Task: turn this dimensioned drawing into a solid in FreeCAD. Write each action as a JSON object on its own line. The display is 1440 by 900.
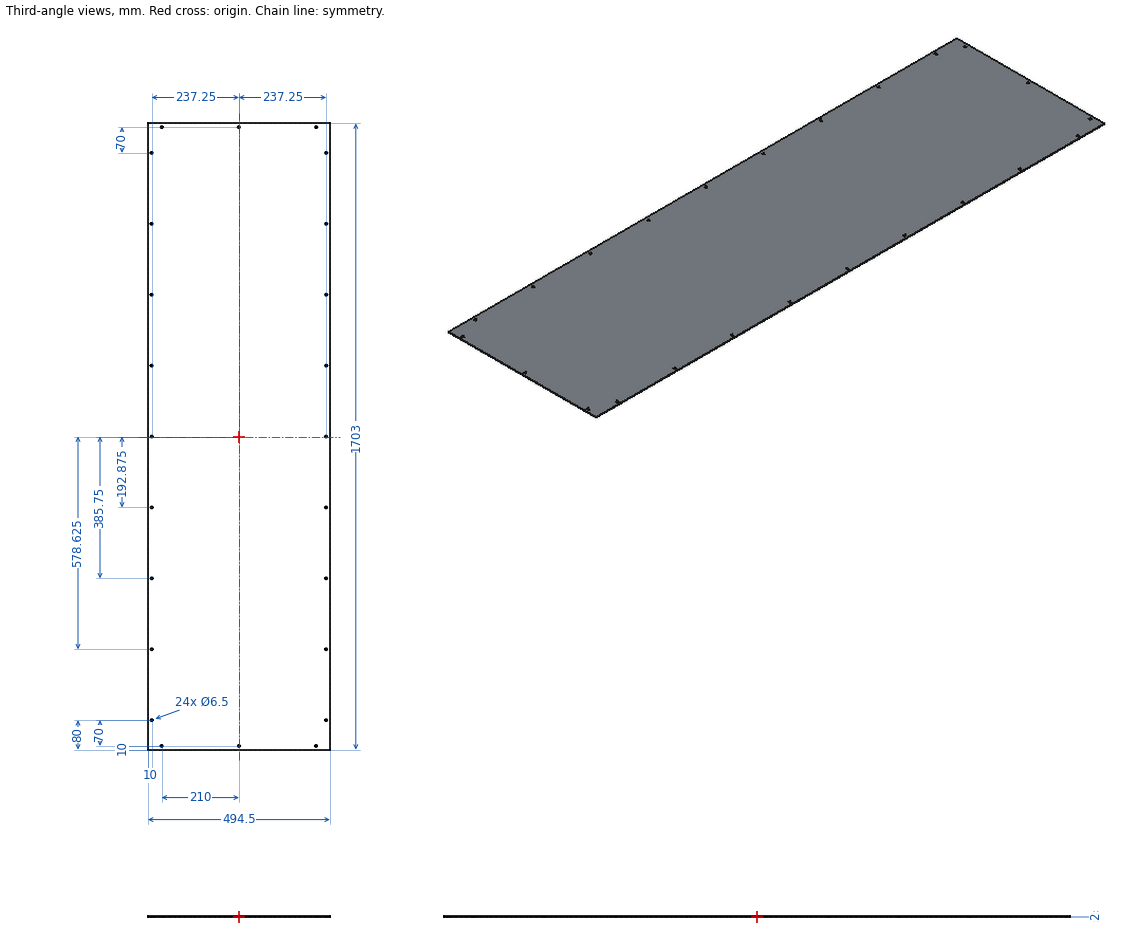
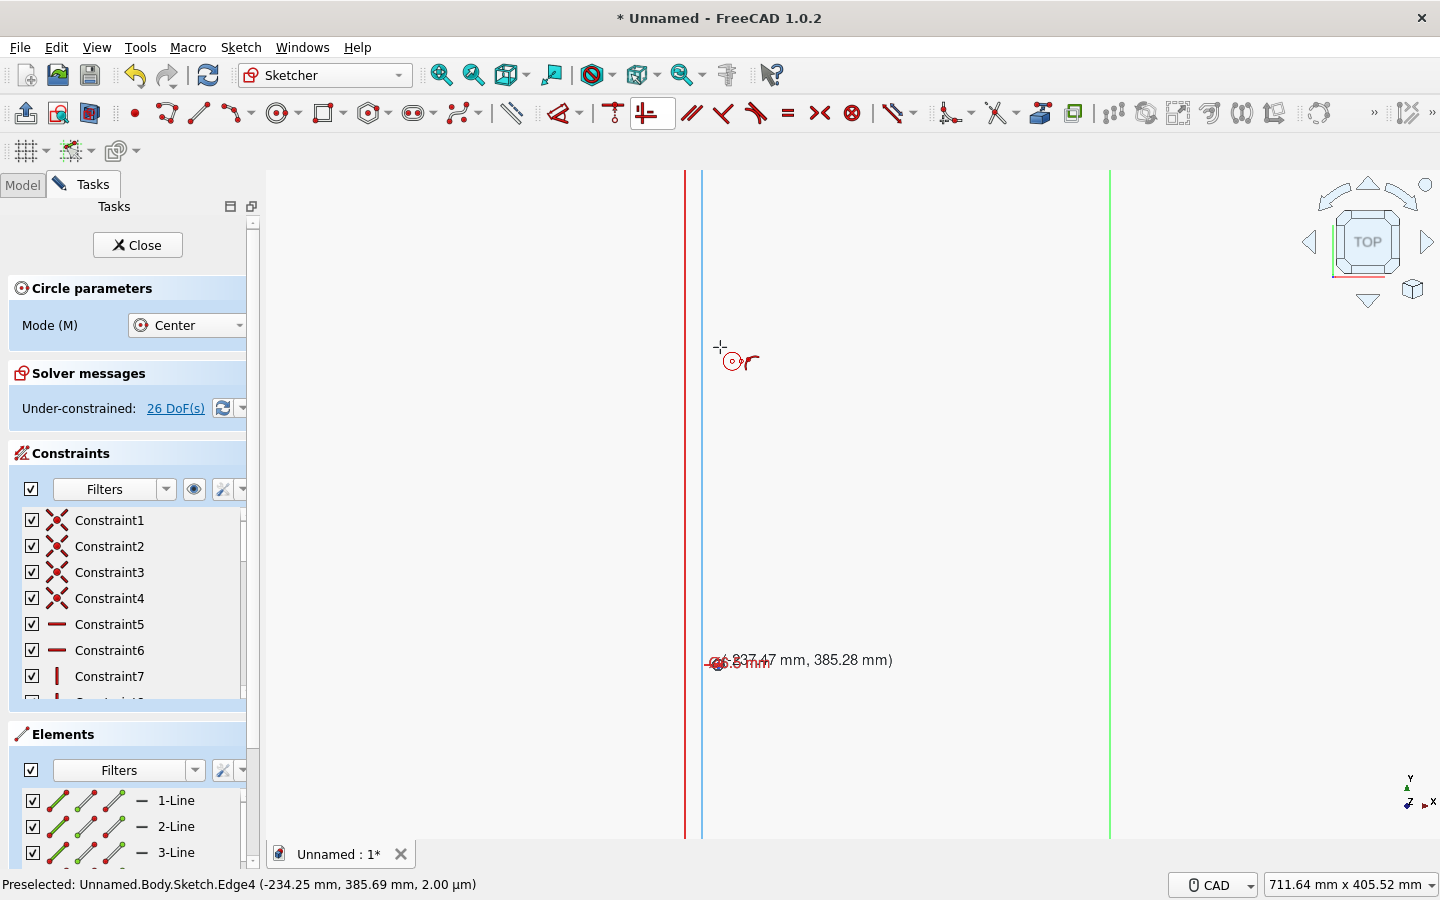
{"action": "left_click", "coordinate": [718, 346]}
{"action": "mouse_move", "coordinate": [722, 342]}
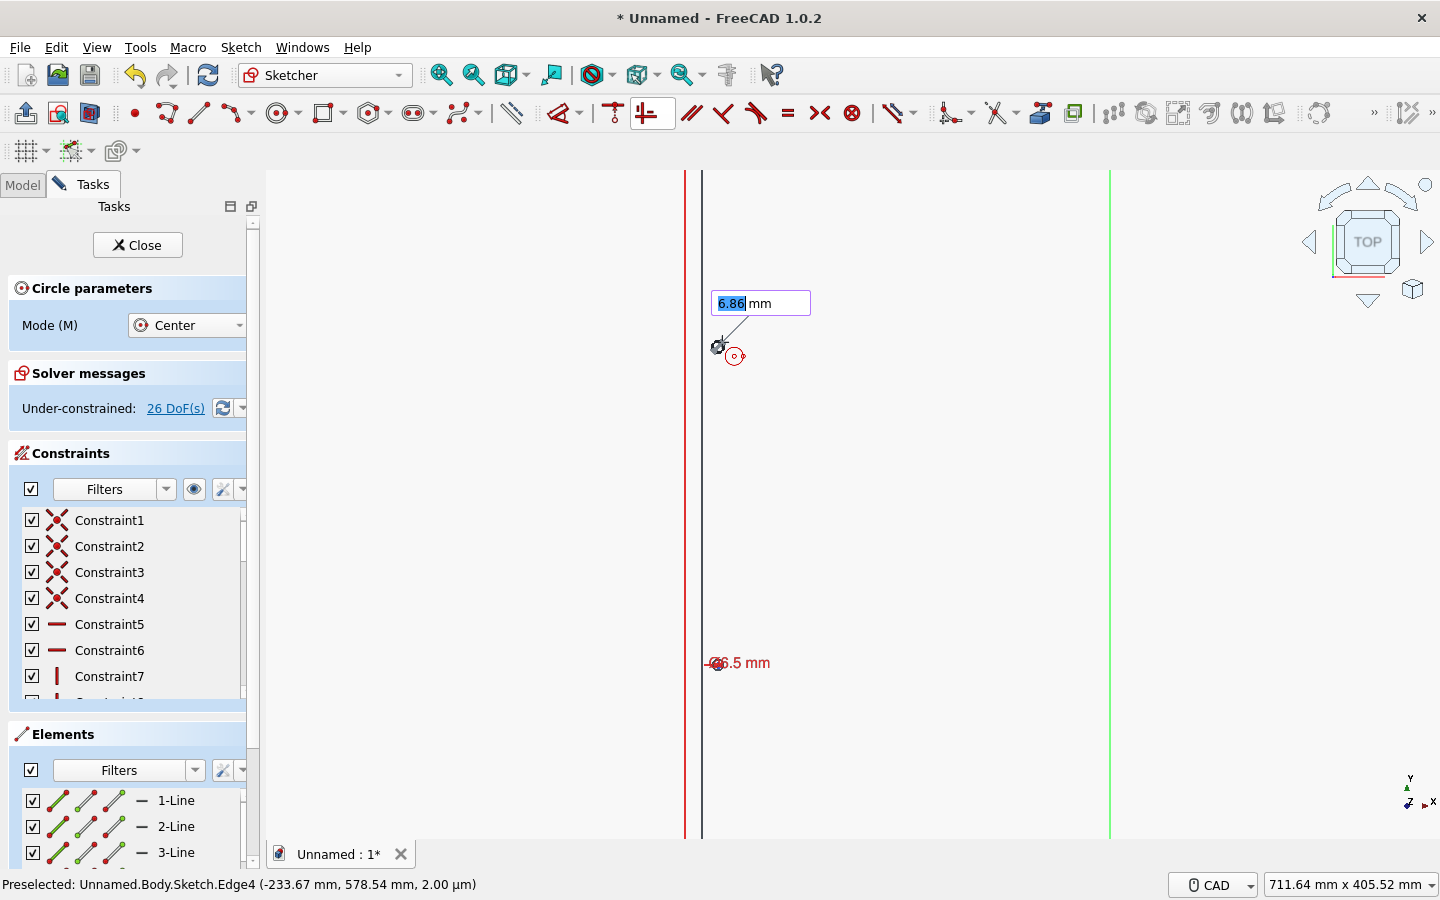
{"action": "type", "text": "6.5"}
{"action": "key", "text": "Return"}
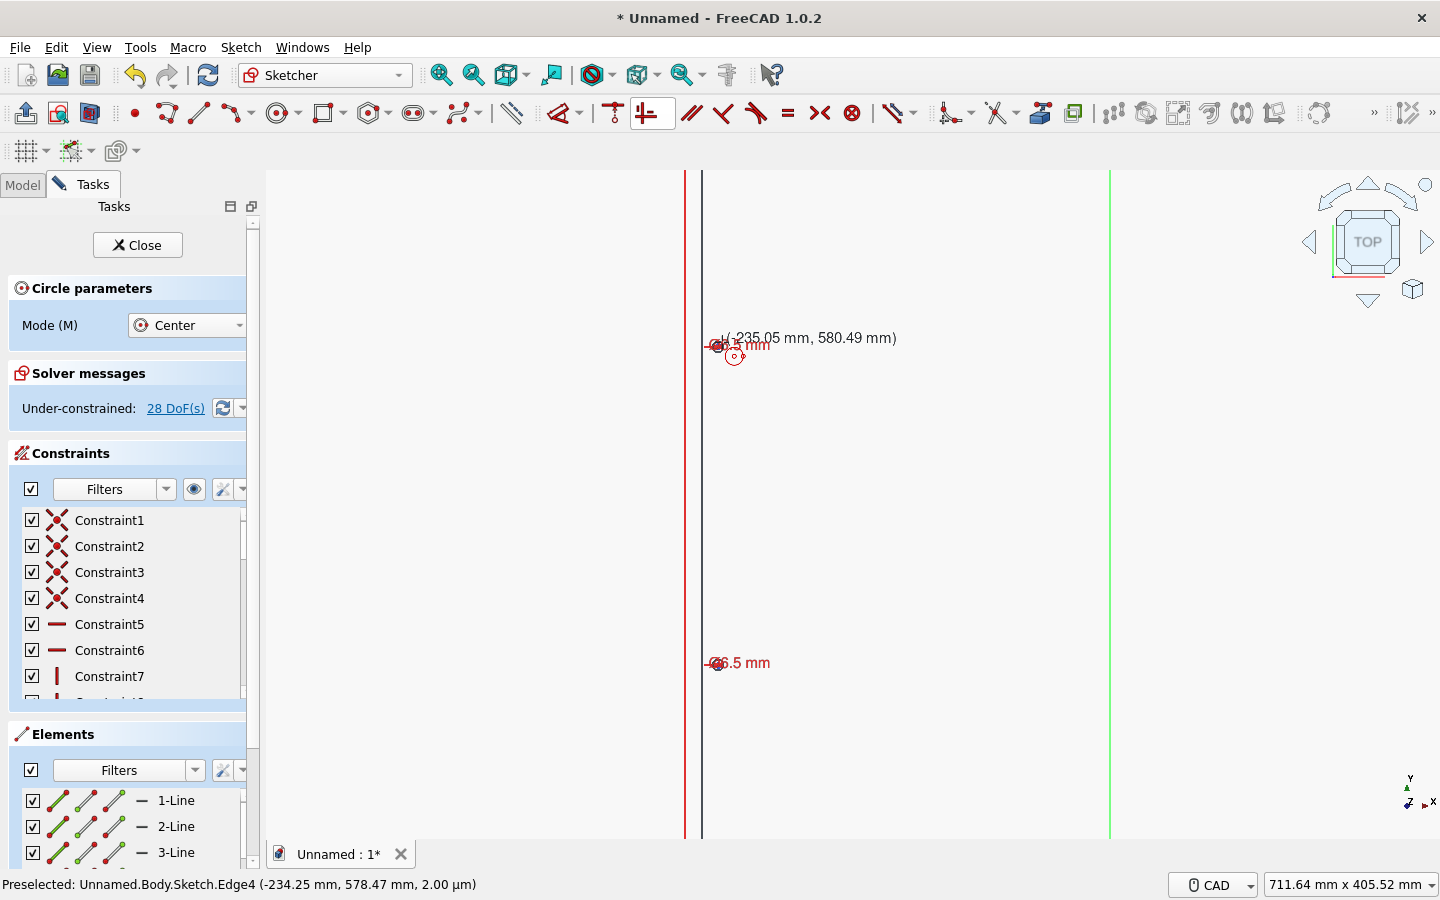
{"action": "scroll", "coordinate": [720, 347], "scroll_direction": "down", "scroll_amount": 9}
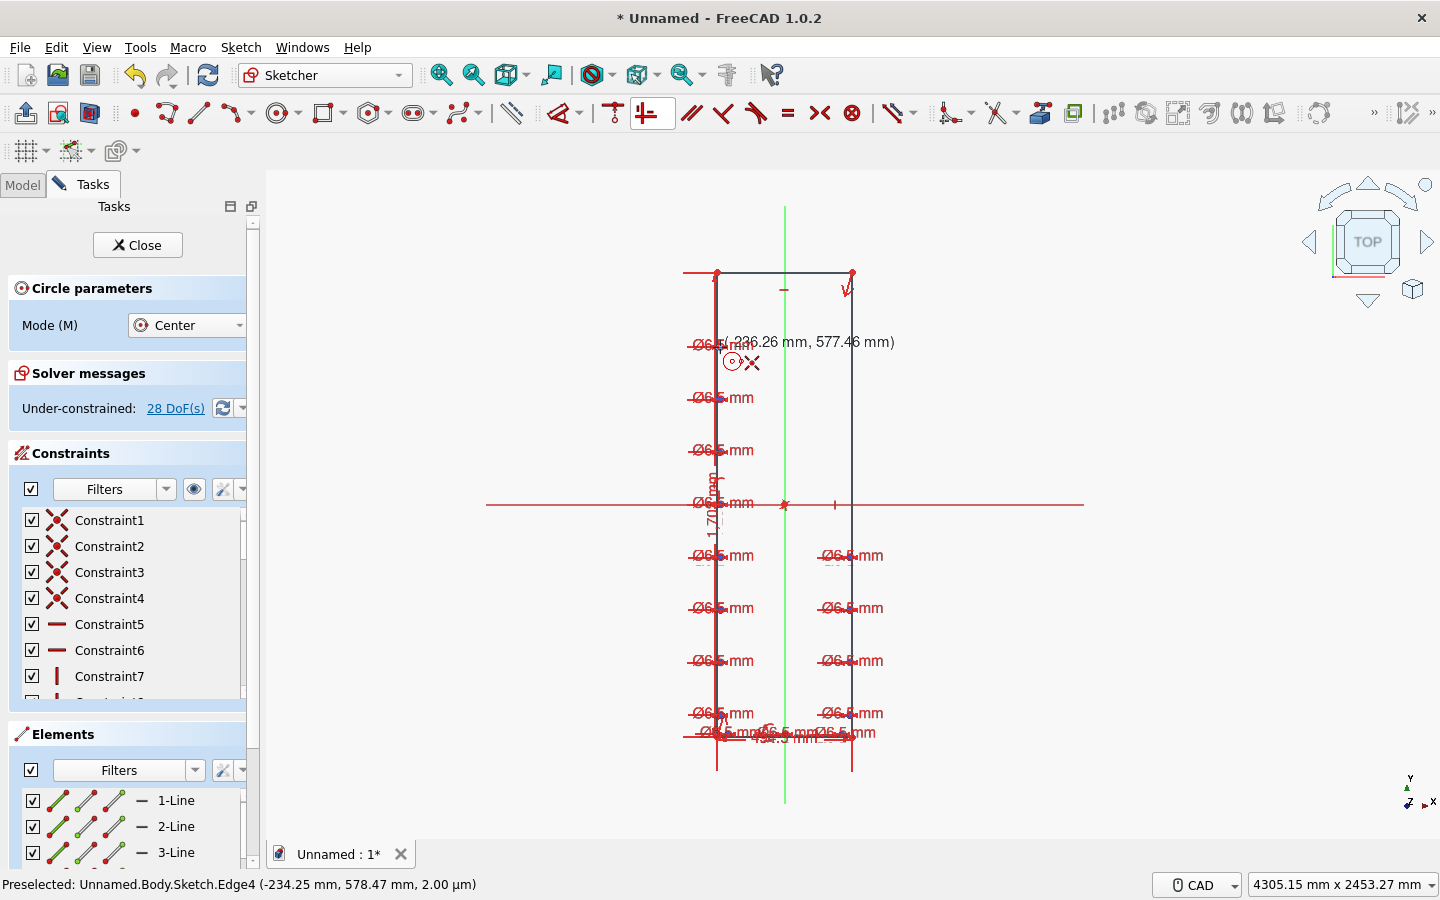
{"action": "scroll", "coordinate": [720, 294], "scroll_direction": "up", "scroll_amount": 17}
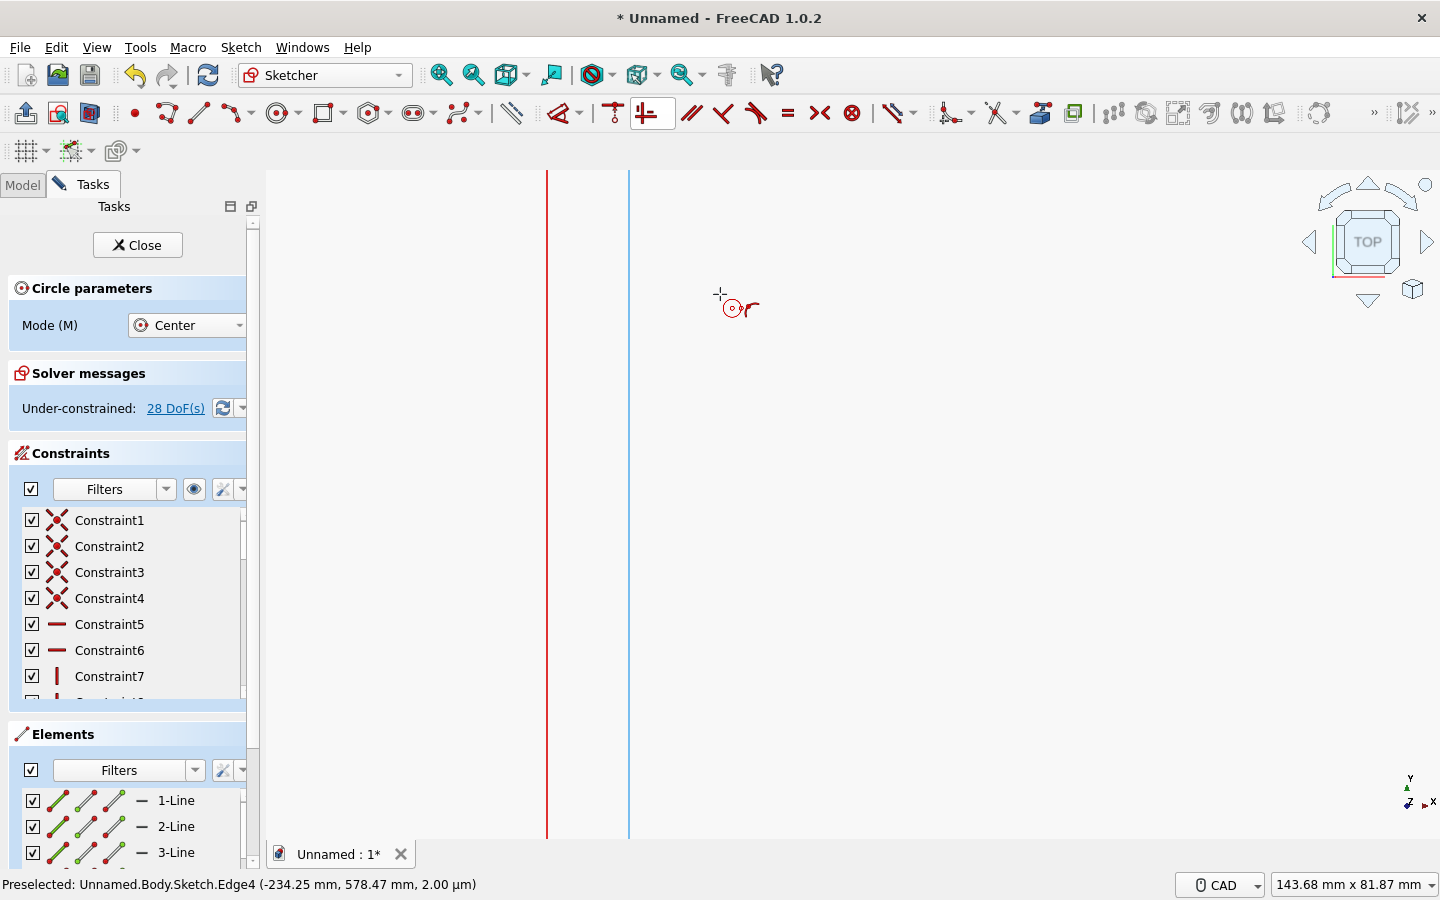
{"action": "scroll", "coordinate": [720, 294], "scroll_direction": "down", "scroll_amount": 17}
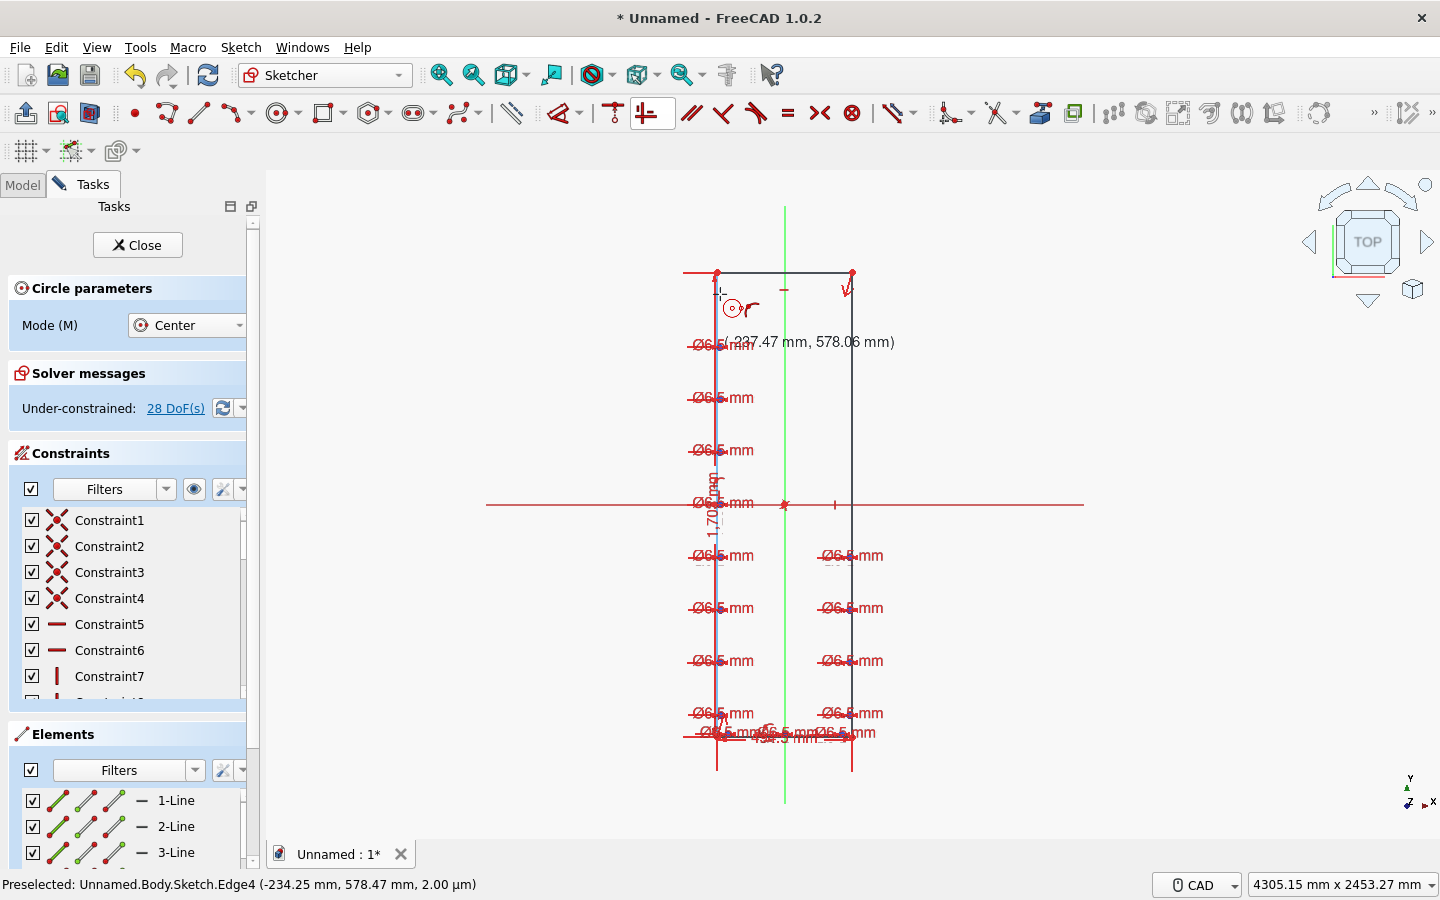
{"action": "scroll", "coordinate": [720, 294], "scroll_direction": "up", "scroll_amount": 9}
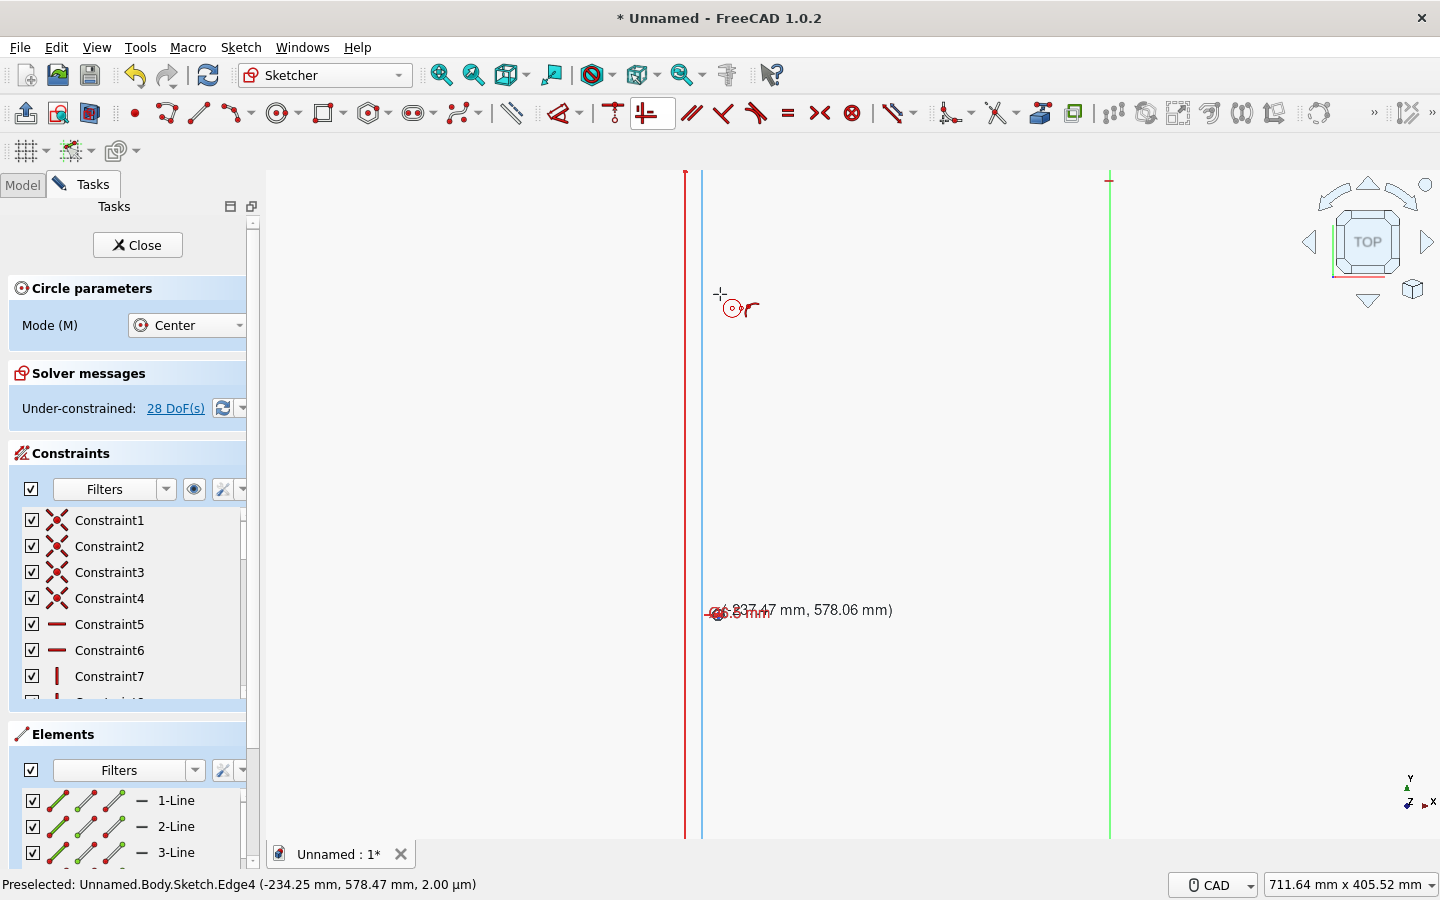
{"action": "left_click", "coordinate": [718, 296]}
{"action": "mouse_move", "coordinate": [722, 292]}